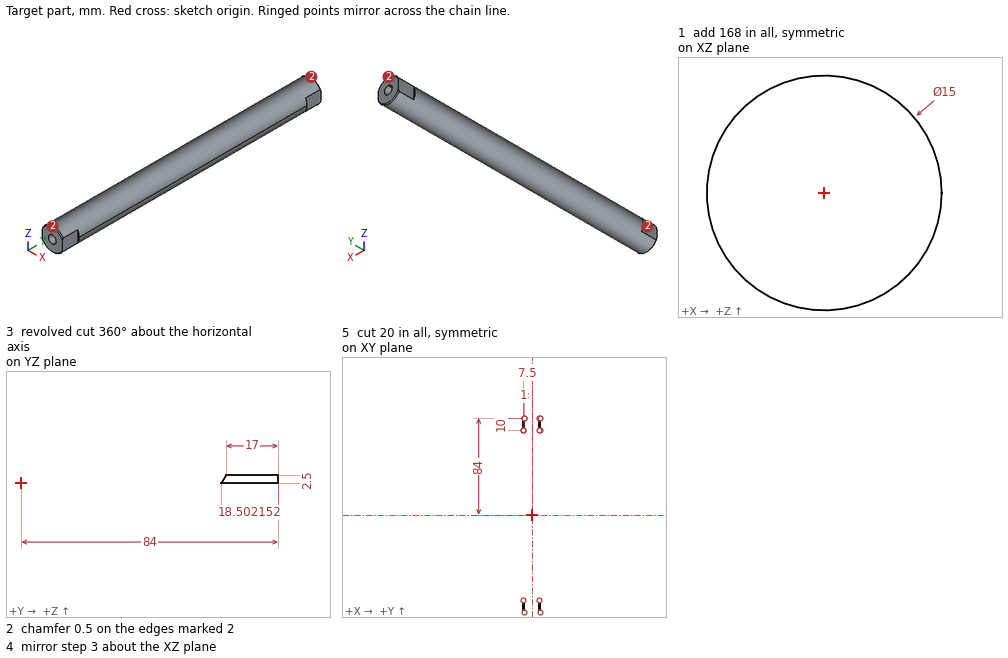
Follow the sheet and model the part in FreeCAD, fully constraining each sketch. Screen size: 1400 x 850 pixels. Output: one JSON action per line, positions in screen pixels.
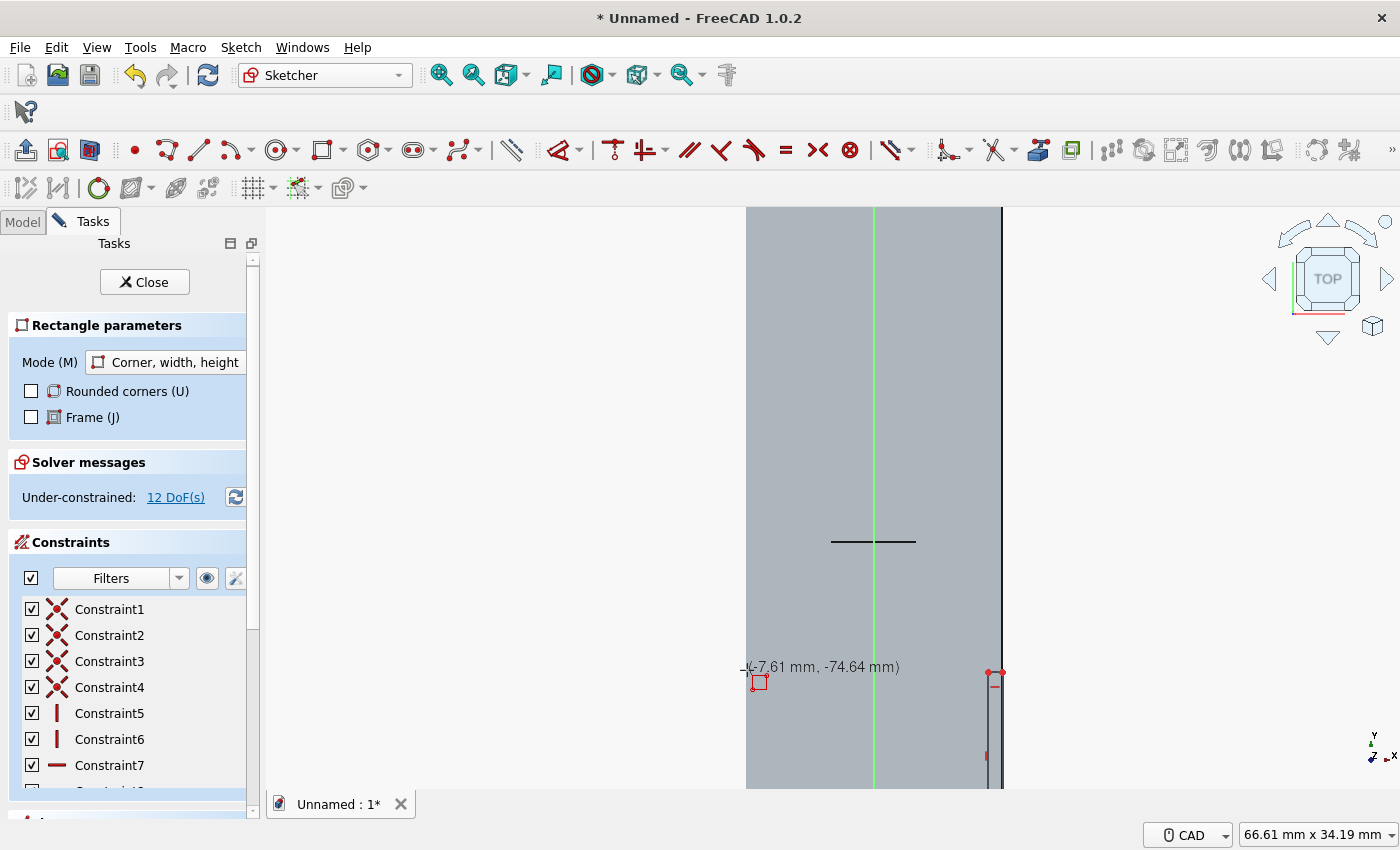
{"action": "scroll", "coordinate": [747, 670], "scroll_direction": "down", "scroll_amount": 10}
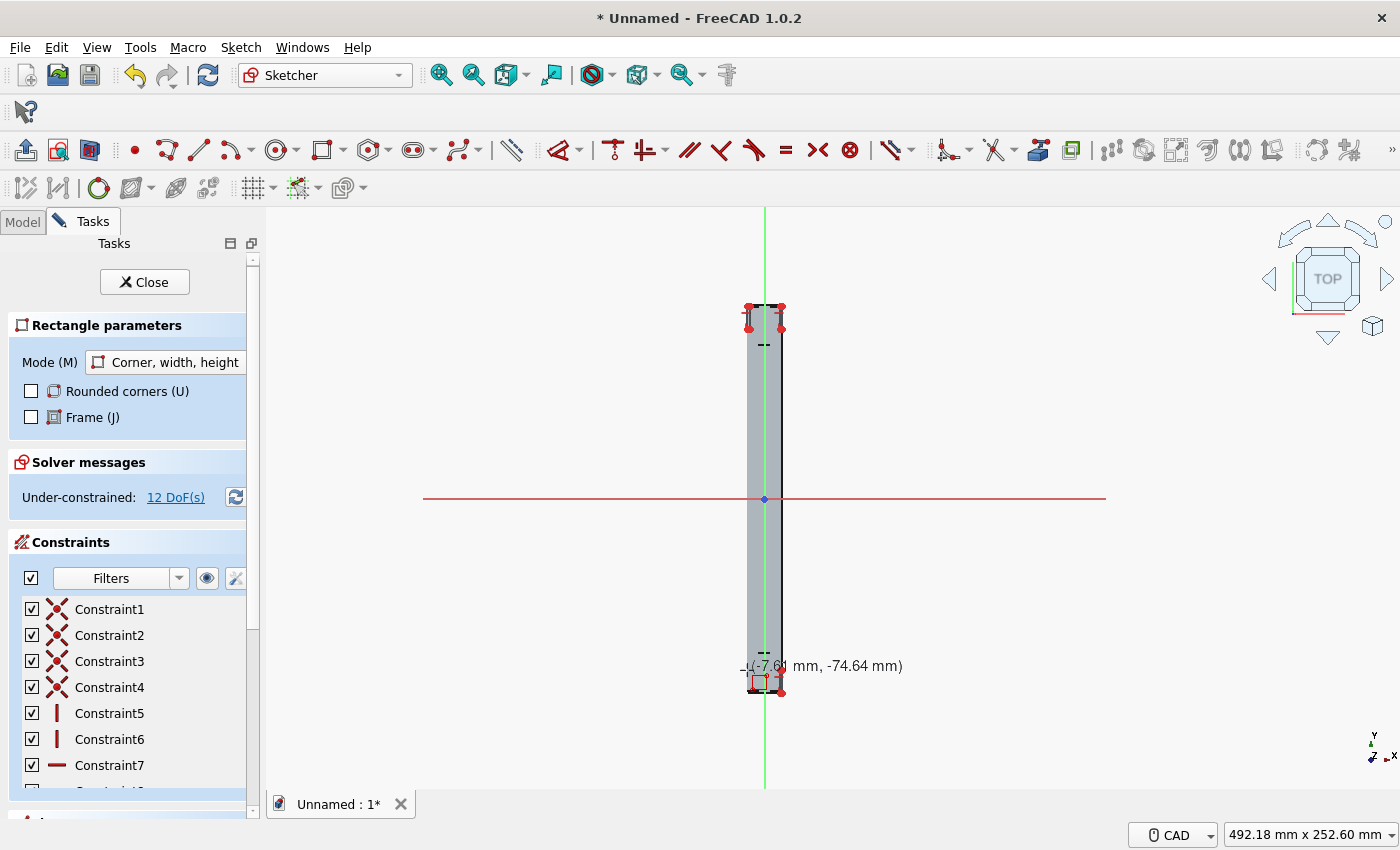
{"action": "left_click", "coordinate": [747, 670]}
{"action": "left_click", "coordinate": [750, 693]}
{"action": "key", "text": "Escape"}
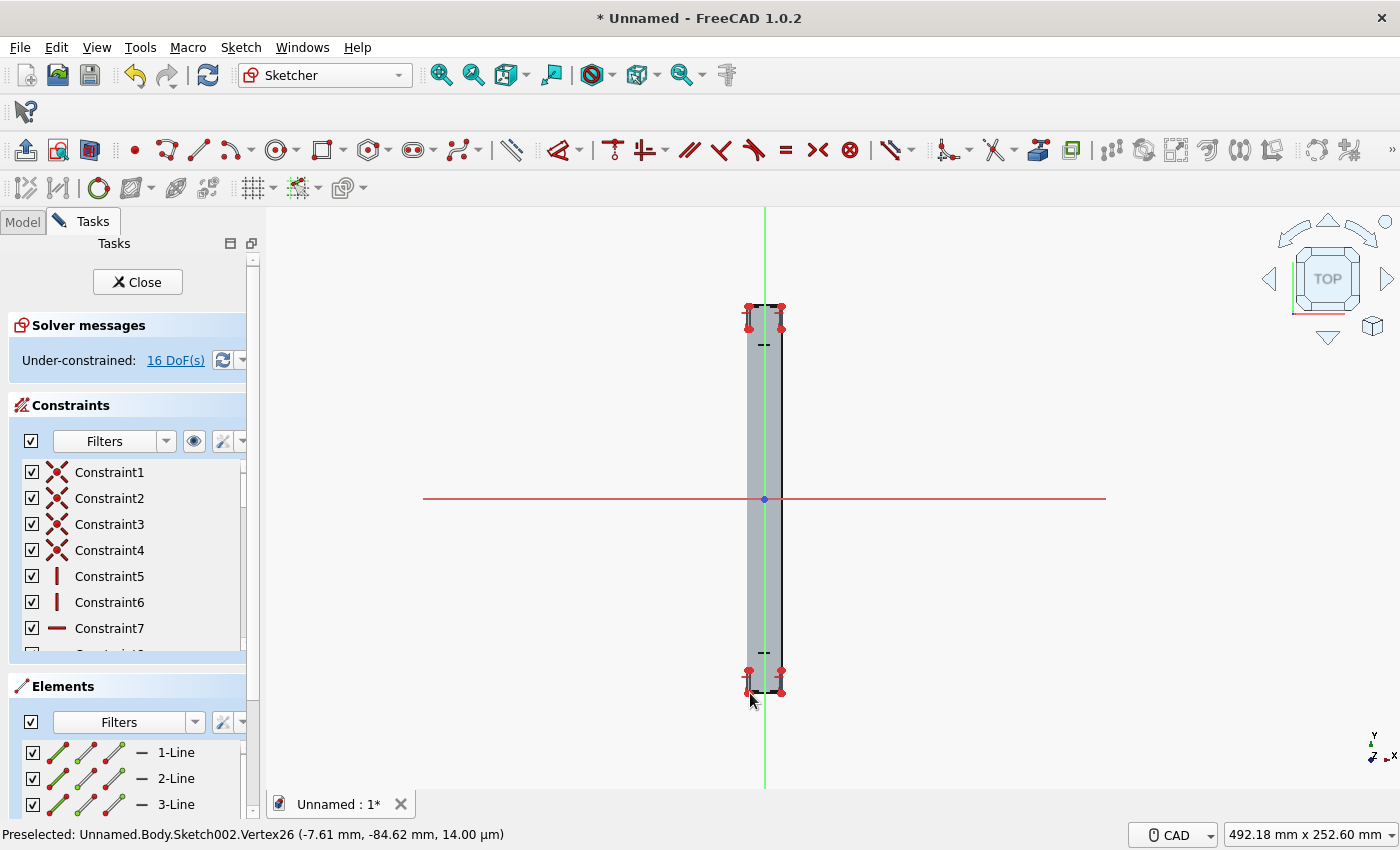
{"action": "scroll", "coordinate": [750, 307], "scroll_direction": "up", "scroll_amount": 8}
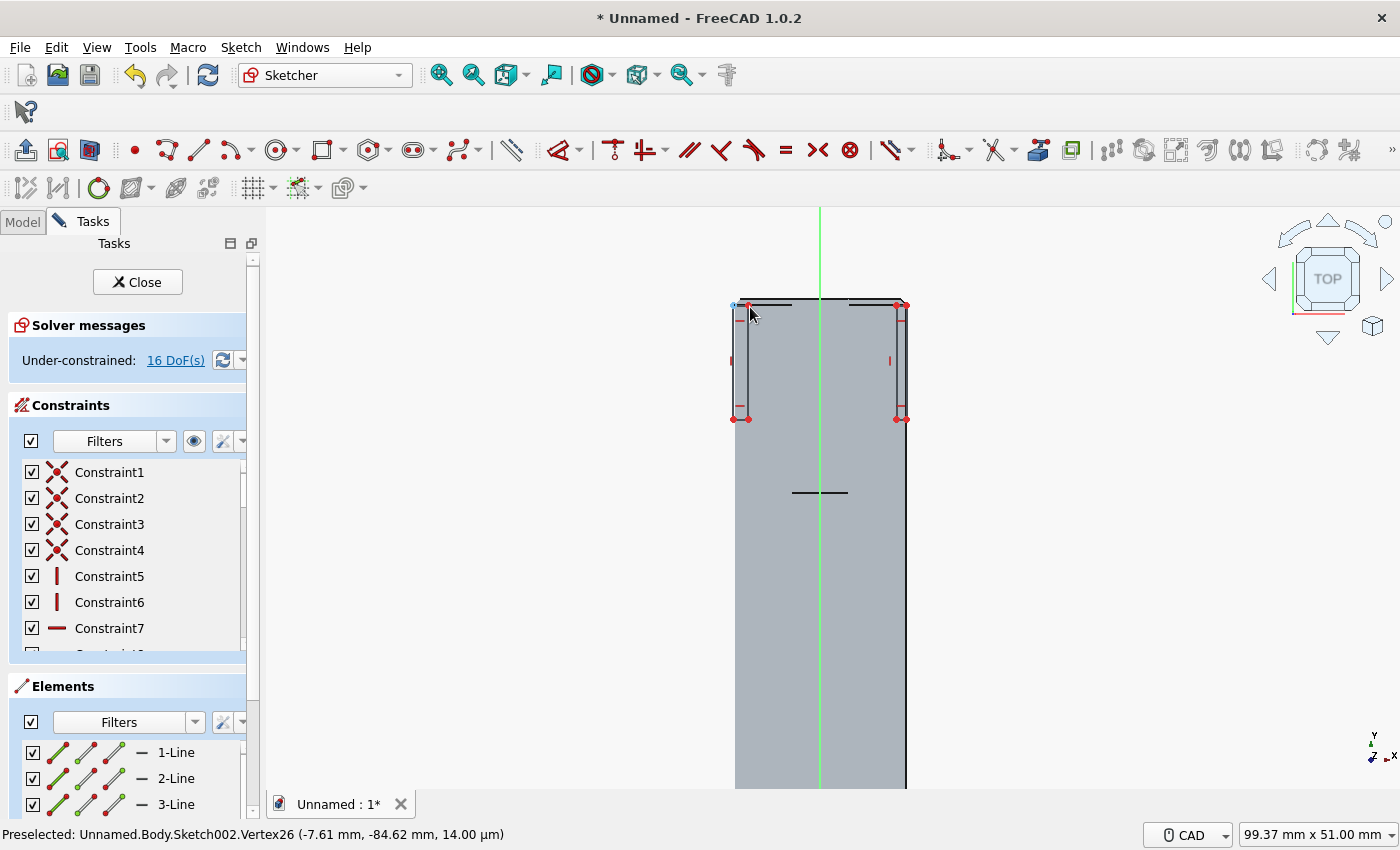
{"action": "left_click", "coordinate": [748, 306]}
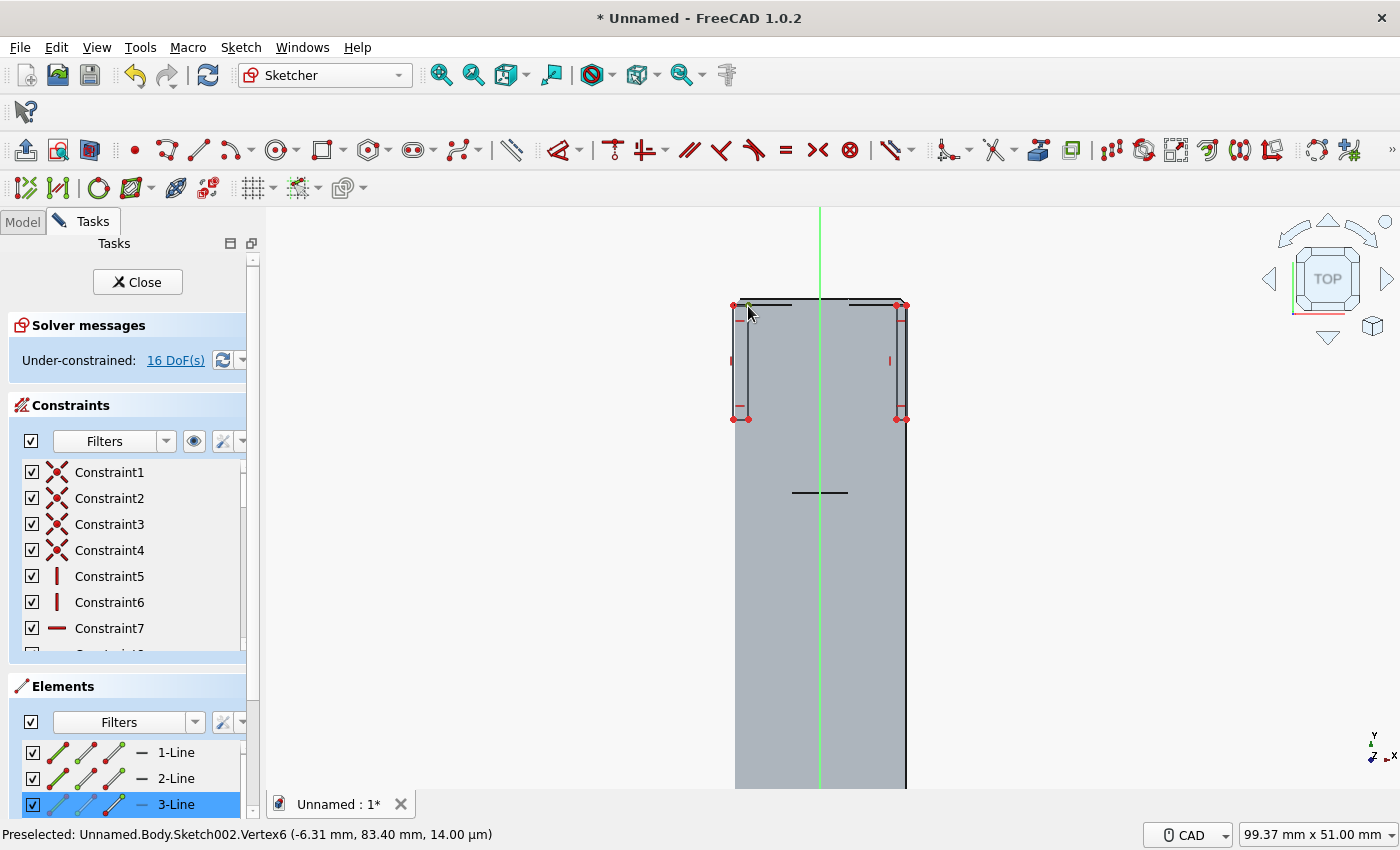
{"action": "scroll", "coordinate": [897, 306], "scroll_direction": "up", "scroll_amount": 2}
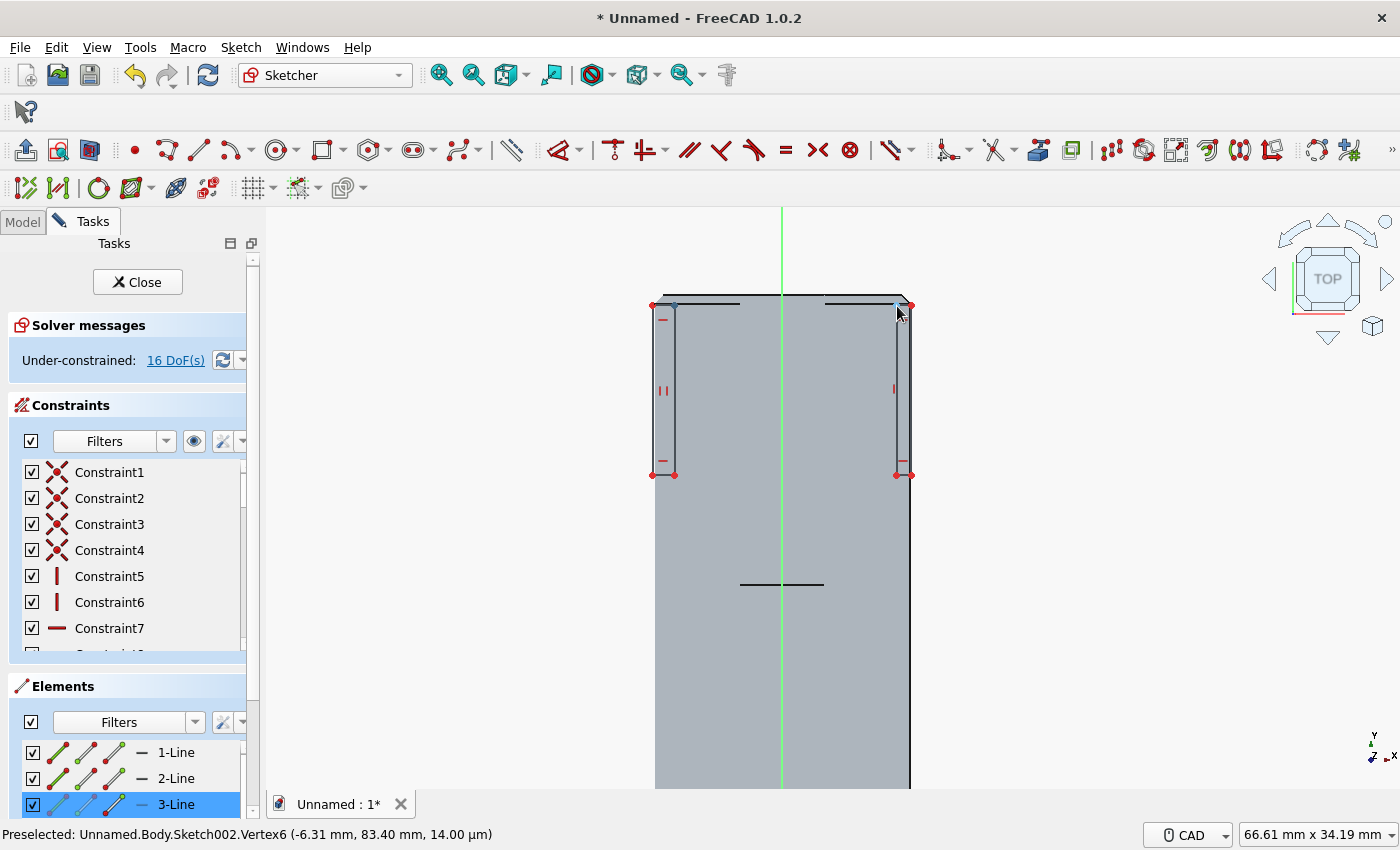
{"action": "left_click", "coordinate": [897, 305]}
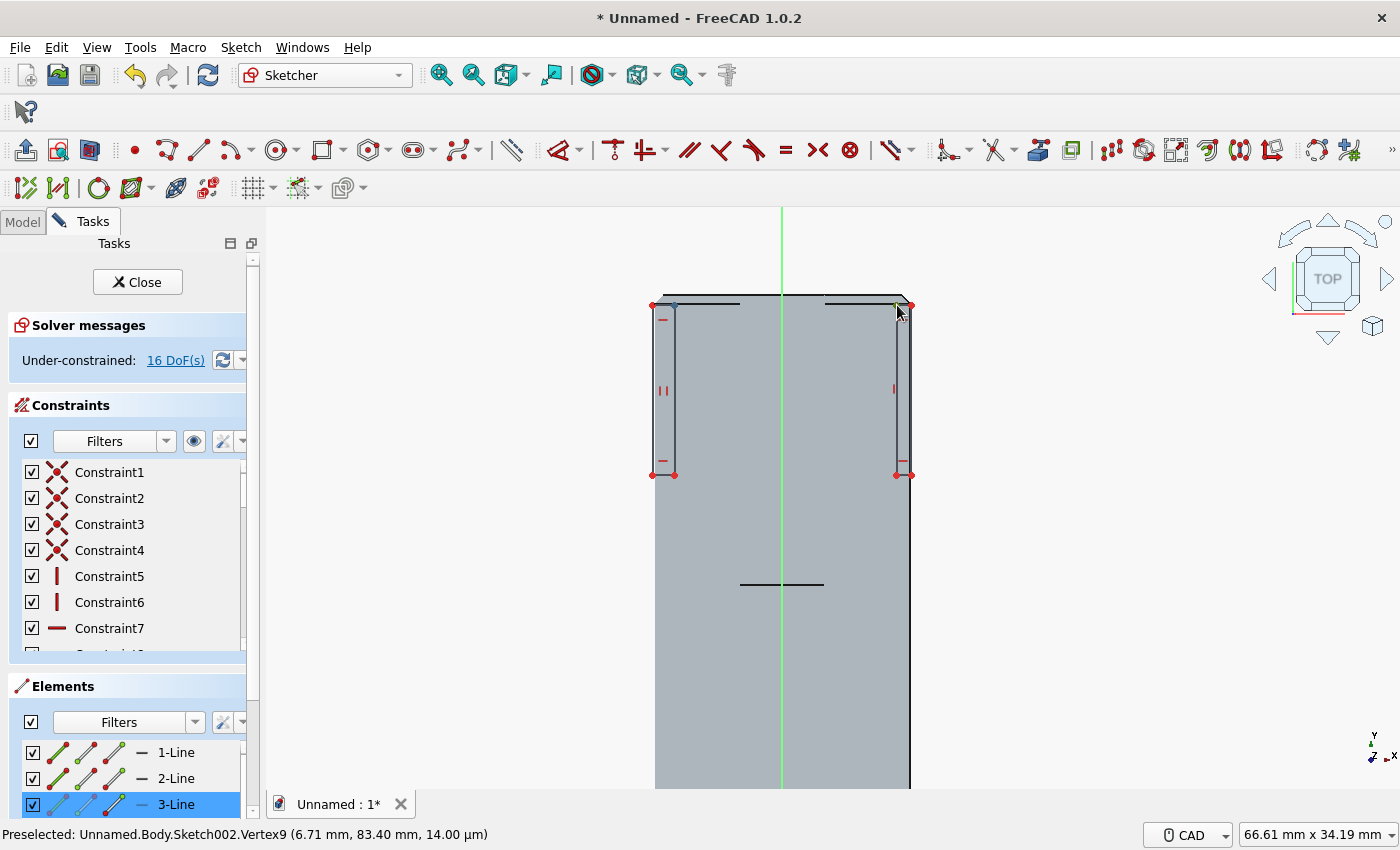
{"action": "left_click", "coordinate": [782, 723]}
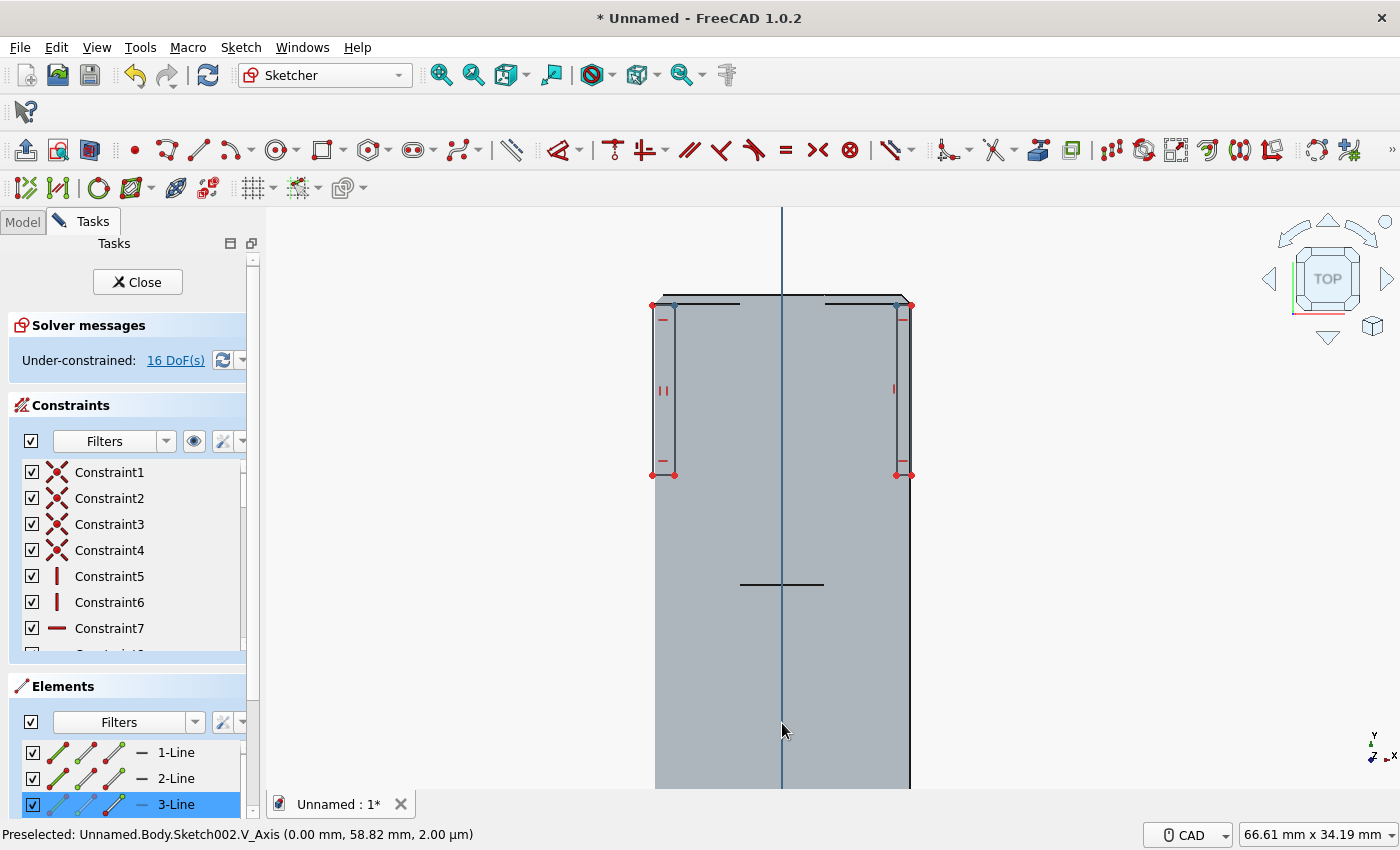
{"action": "left_click", "coordinate": [818, 150]}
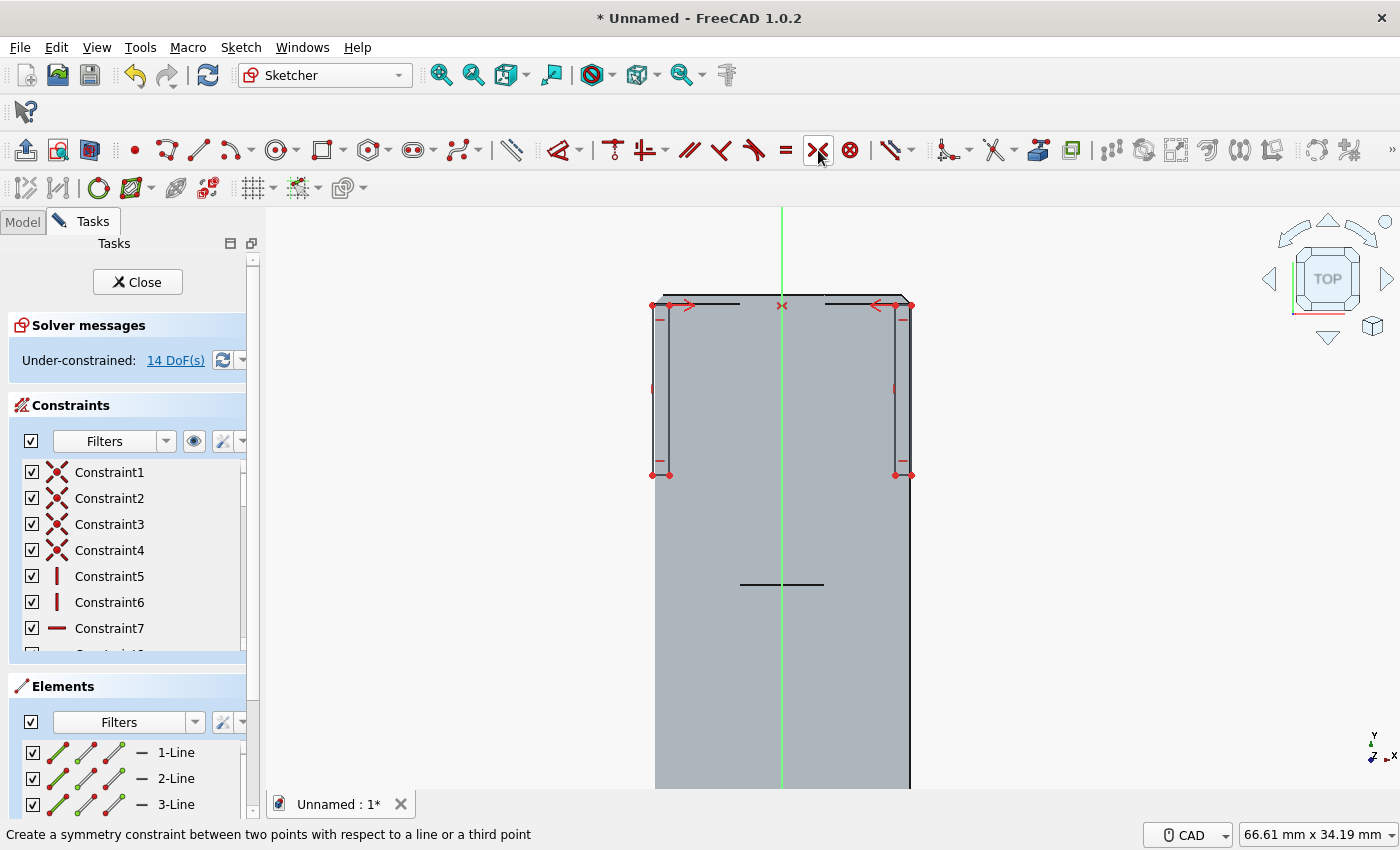
{"action": "left_click", "coordinate": [653, 475]}